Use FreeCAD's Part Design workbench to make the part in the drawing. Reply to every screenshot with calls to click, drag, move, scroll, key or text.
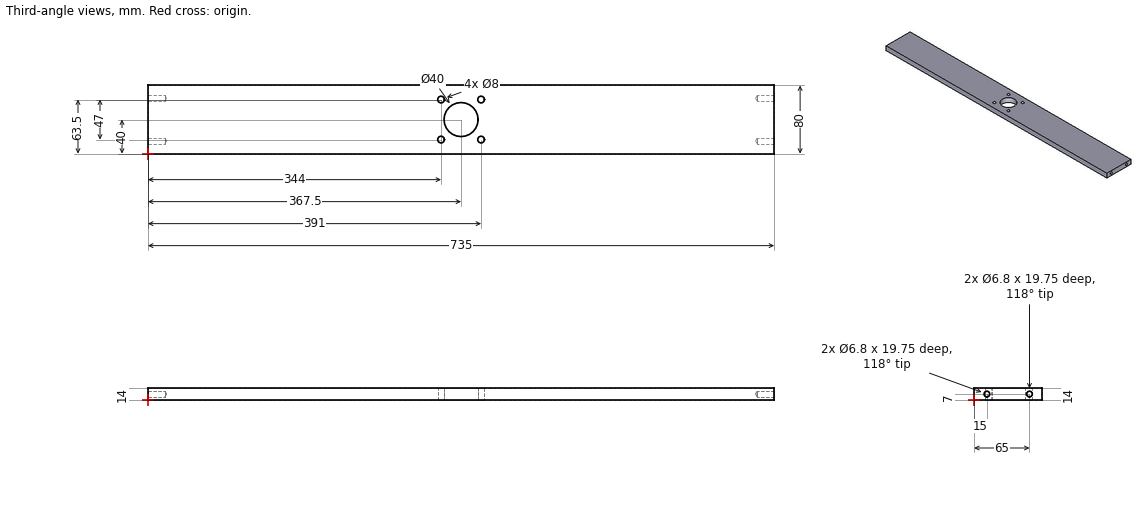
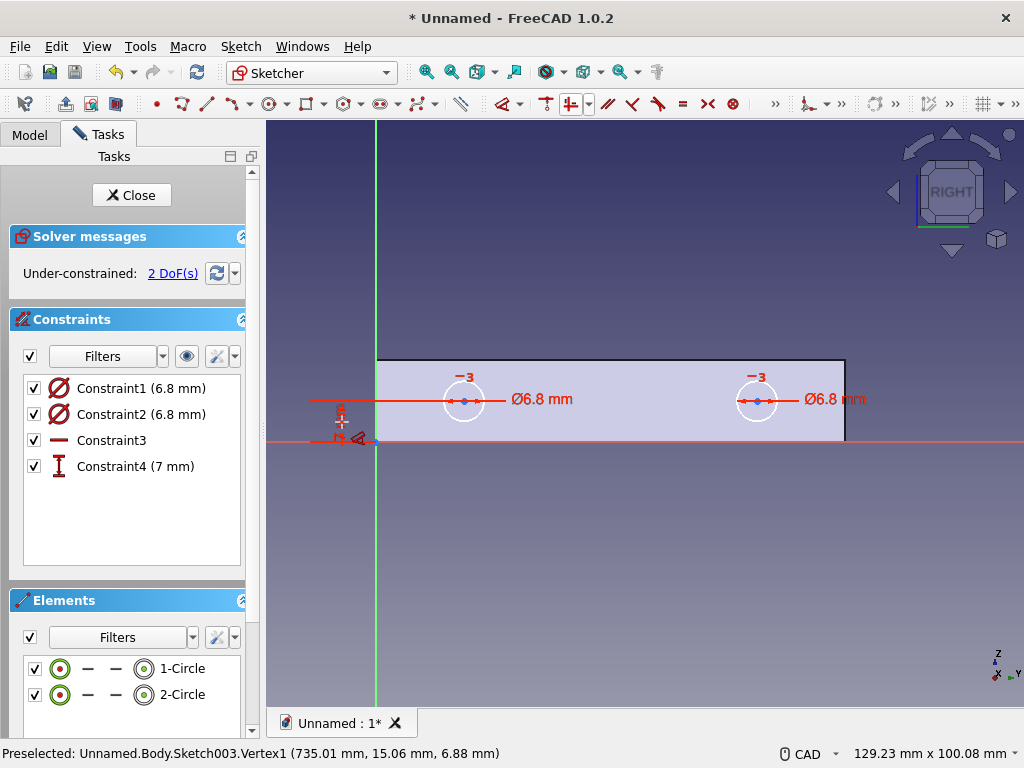
click(464, 401)
click(420, 476)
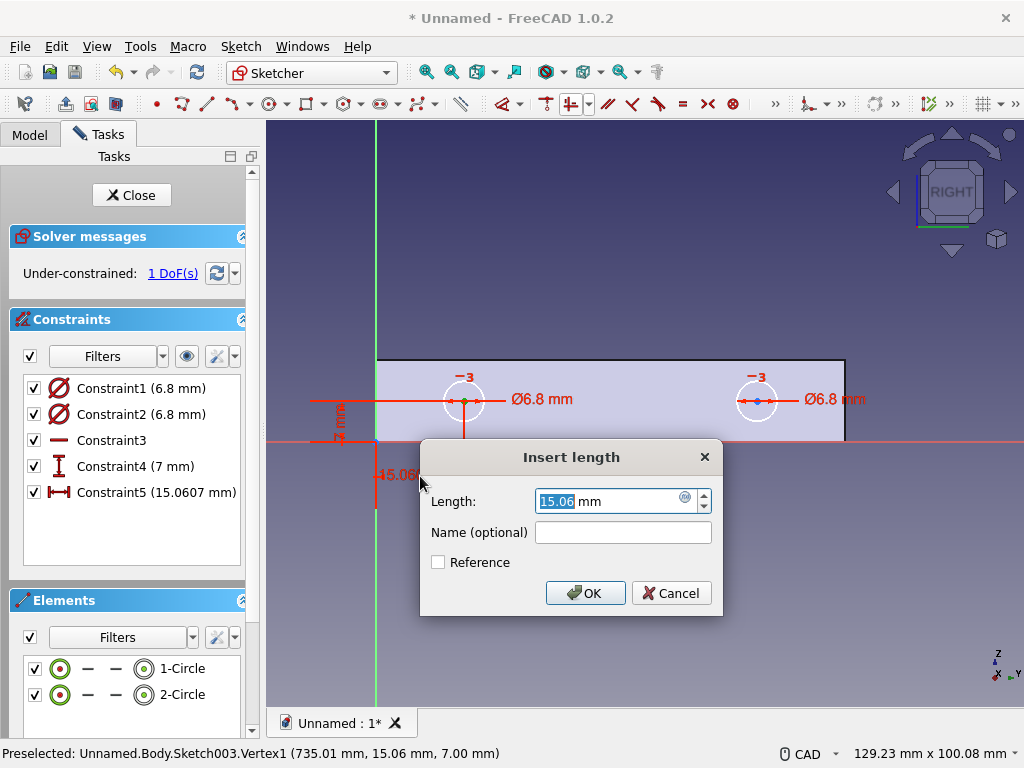
text(15)
key(Return)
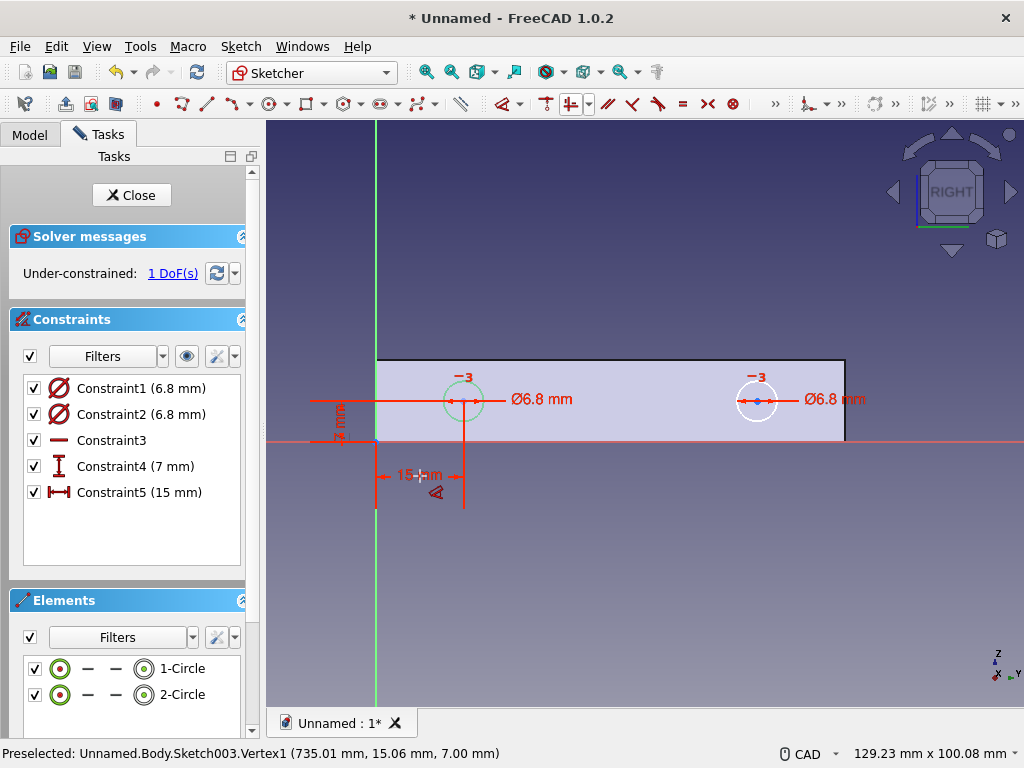
click(757, 401)
click(566, 476)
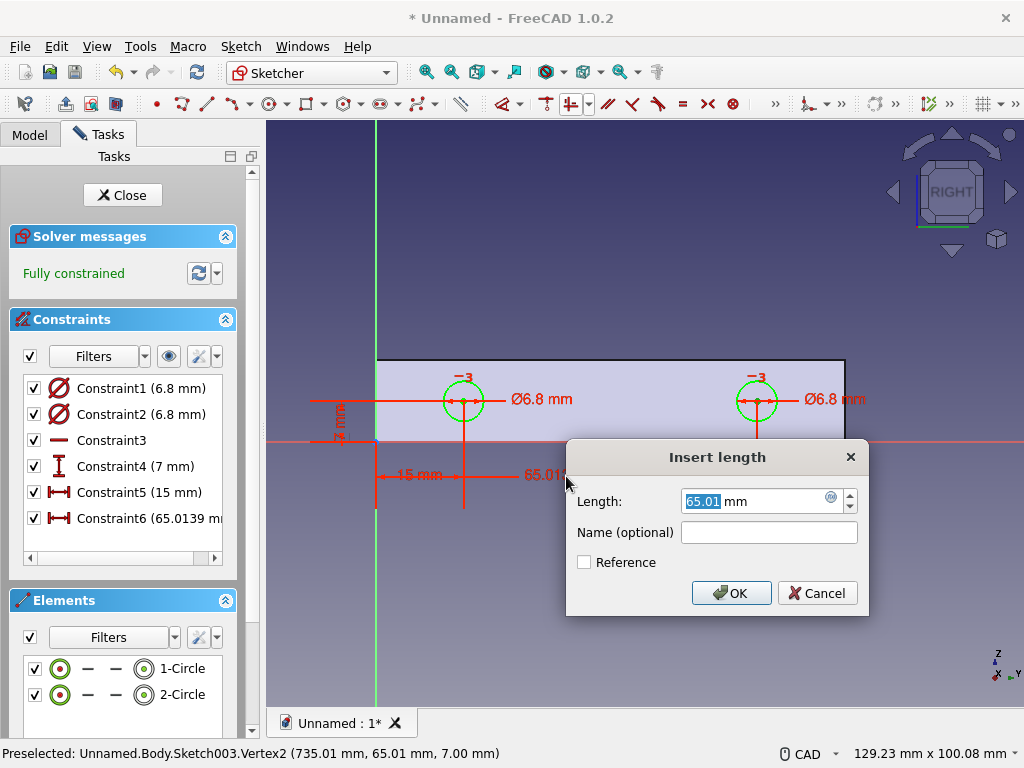
text(65)
key(Return)
key(Escape)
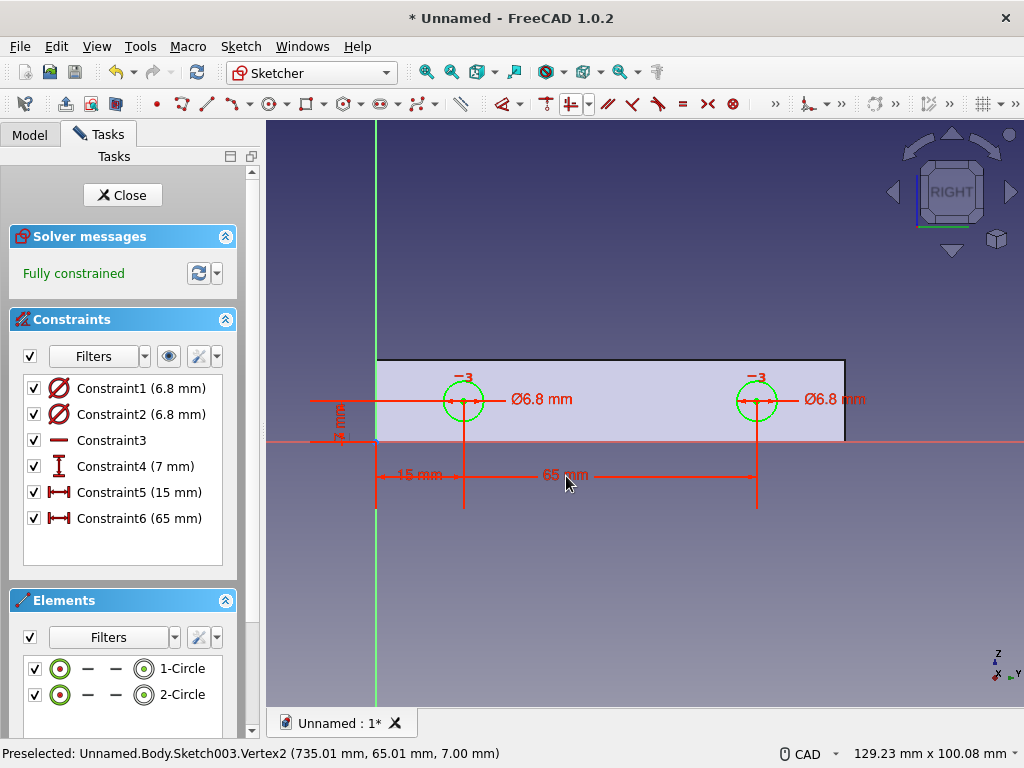
click(123, 195)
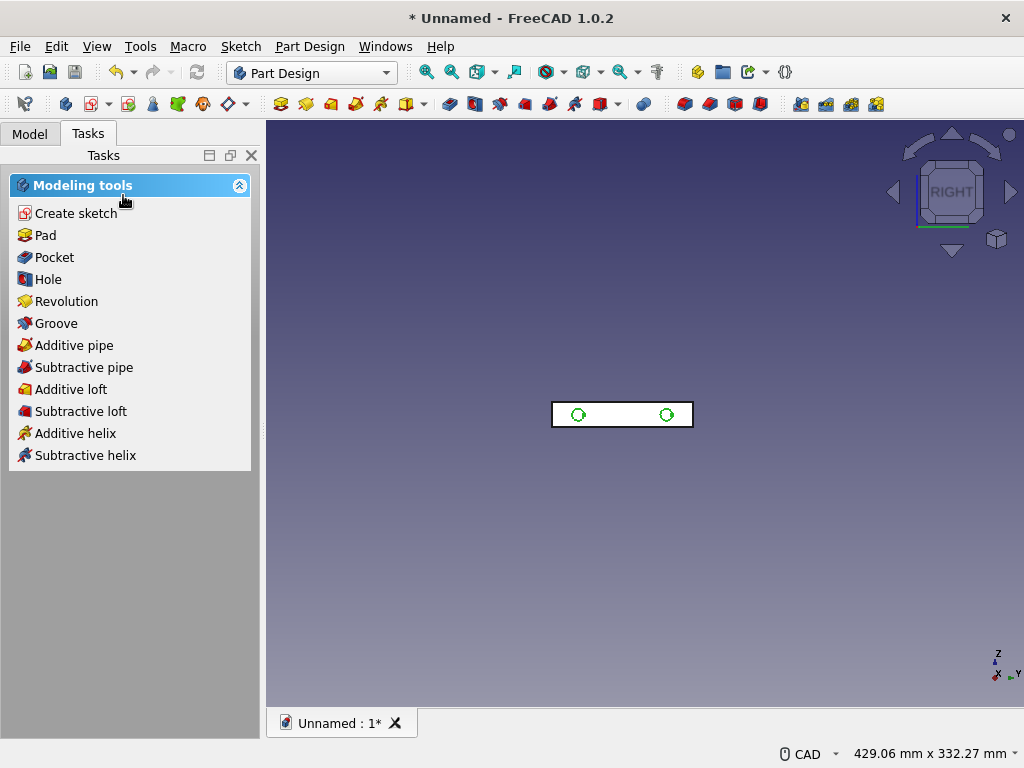
click(475, 104)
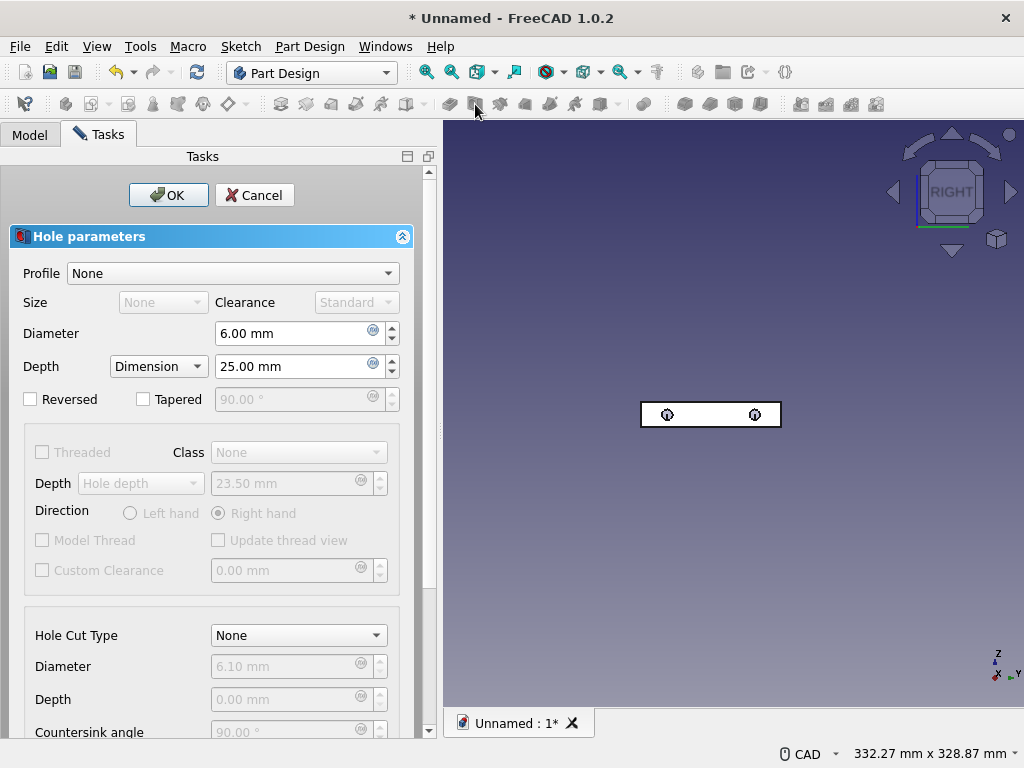
triple_click(300, 334)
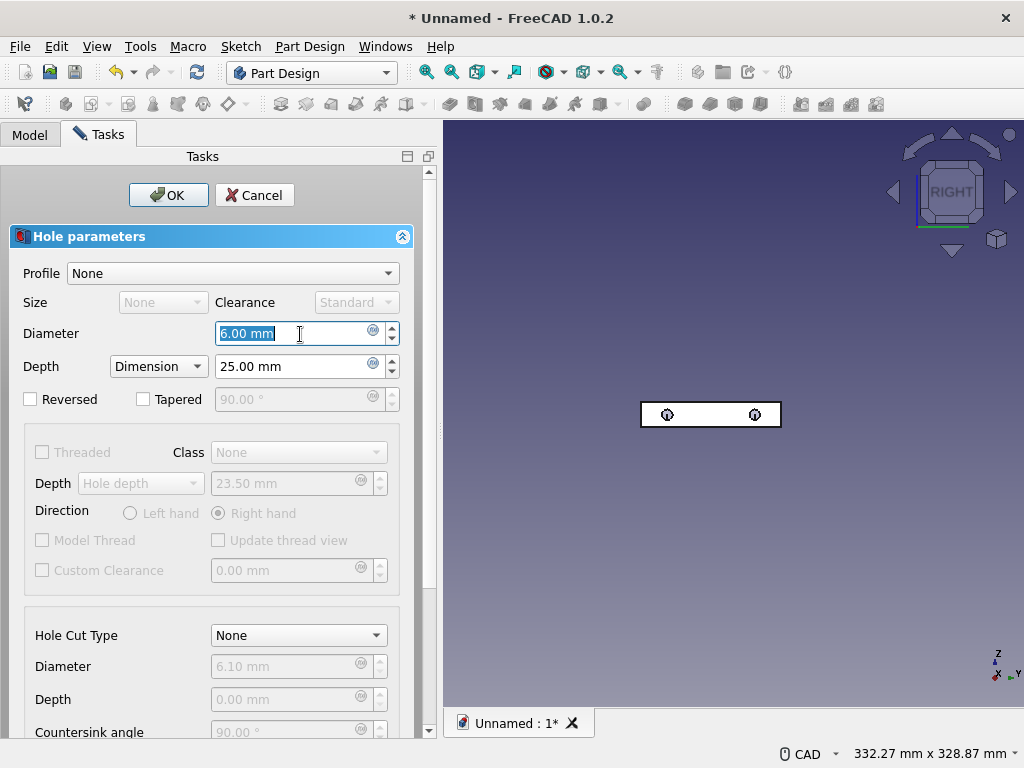
text(6.8)
key(Tab)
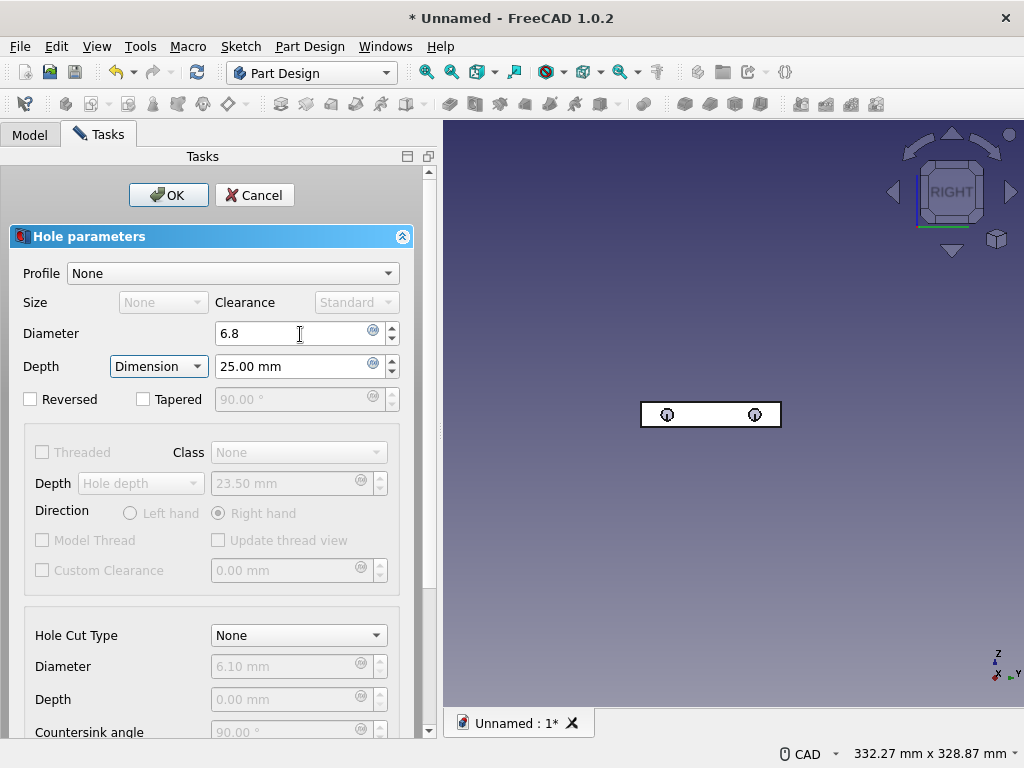
triple_click(300, 366)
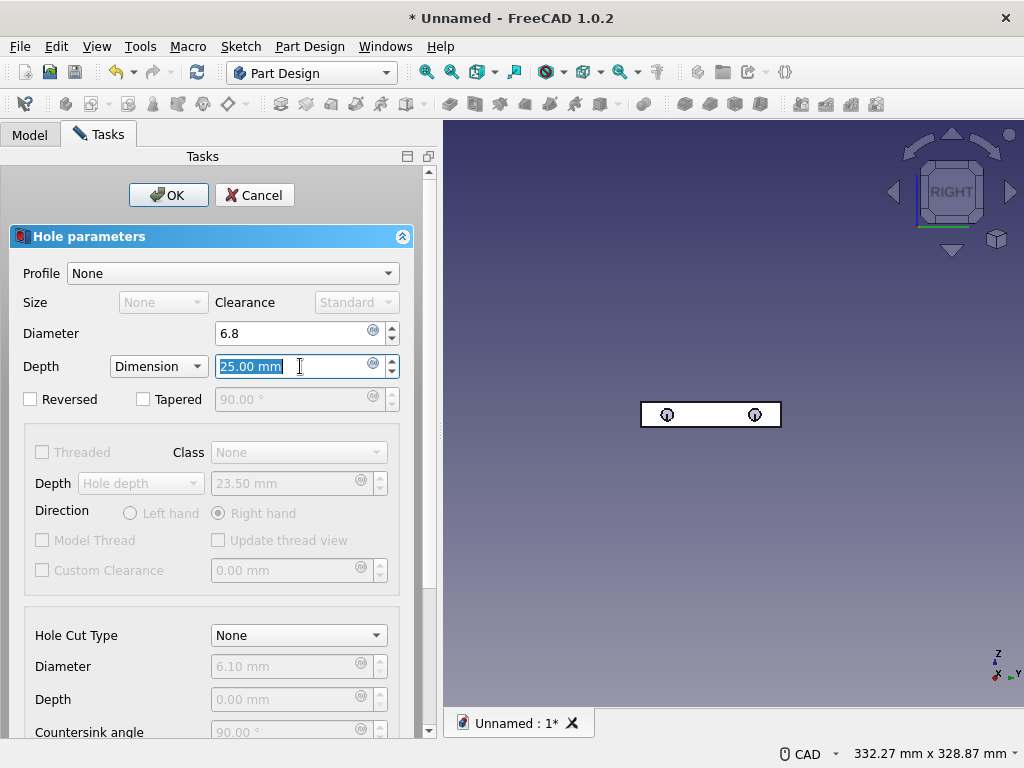
text(19.75)
key(Tab)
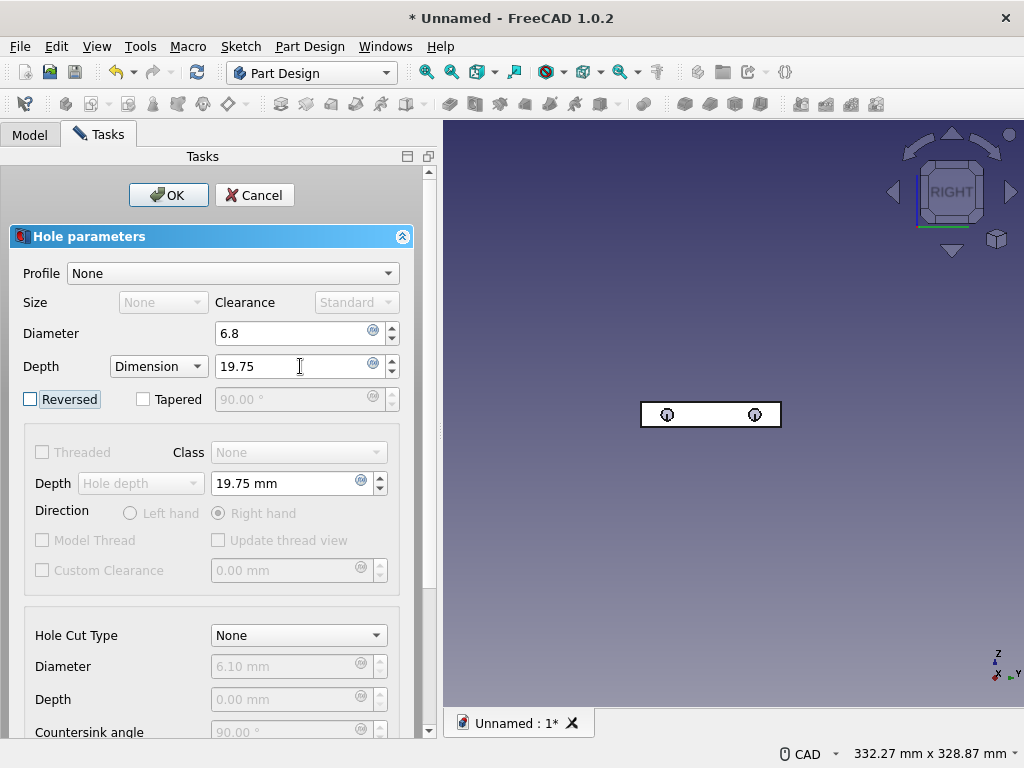
click(169, 195)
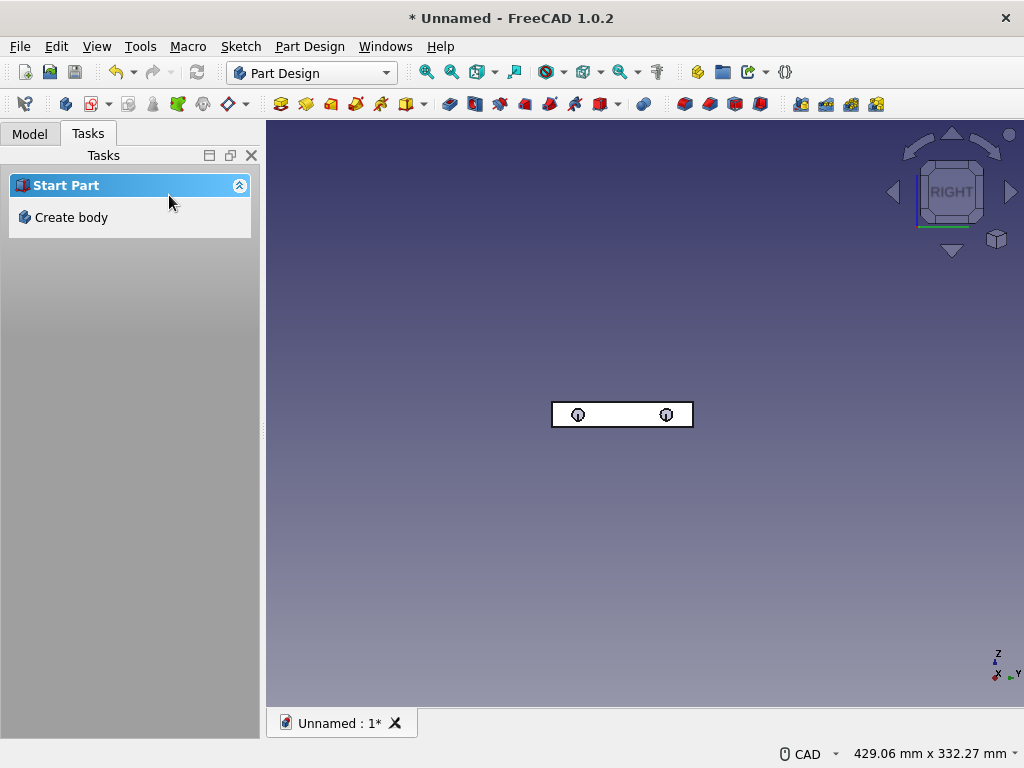
key(0)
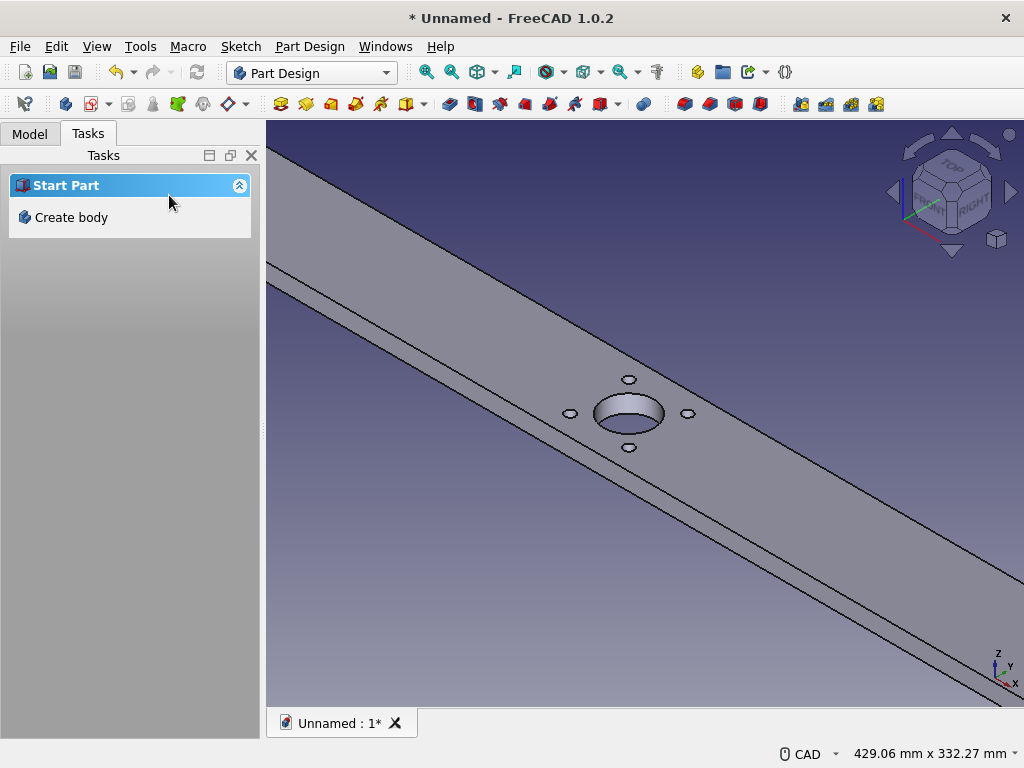
key(v)
key(f)